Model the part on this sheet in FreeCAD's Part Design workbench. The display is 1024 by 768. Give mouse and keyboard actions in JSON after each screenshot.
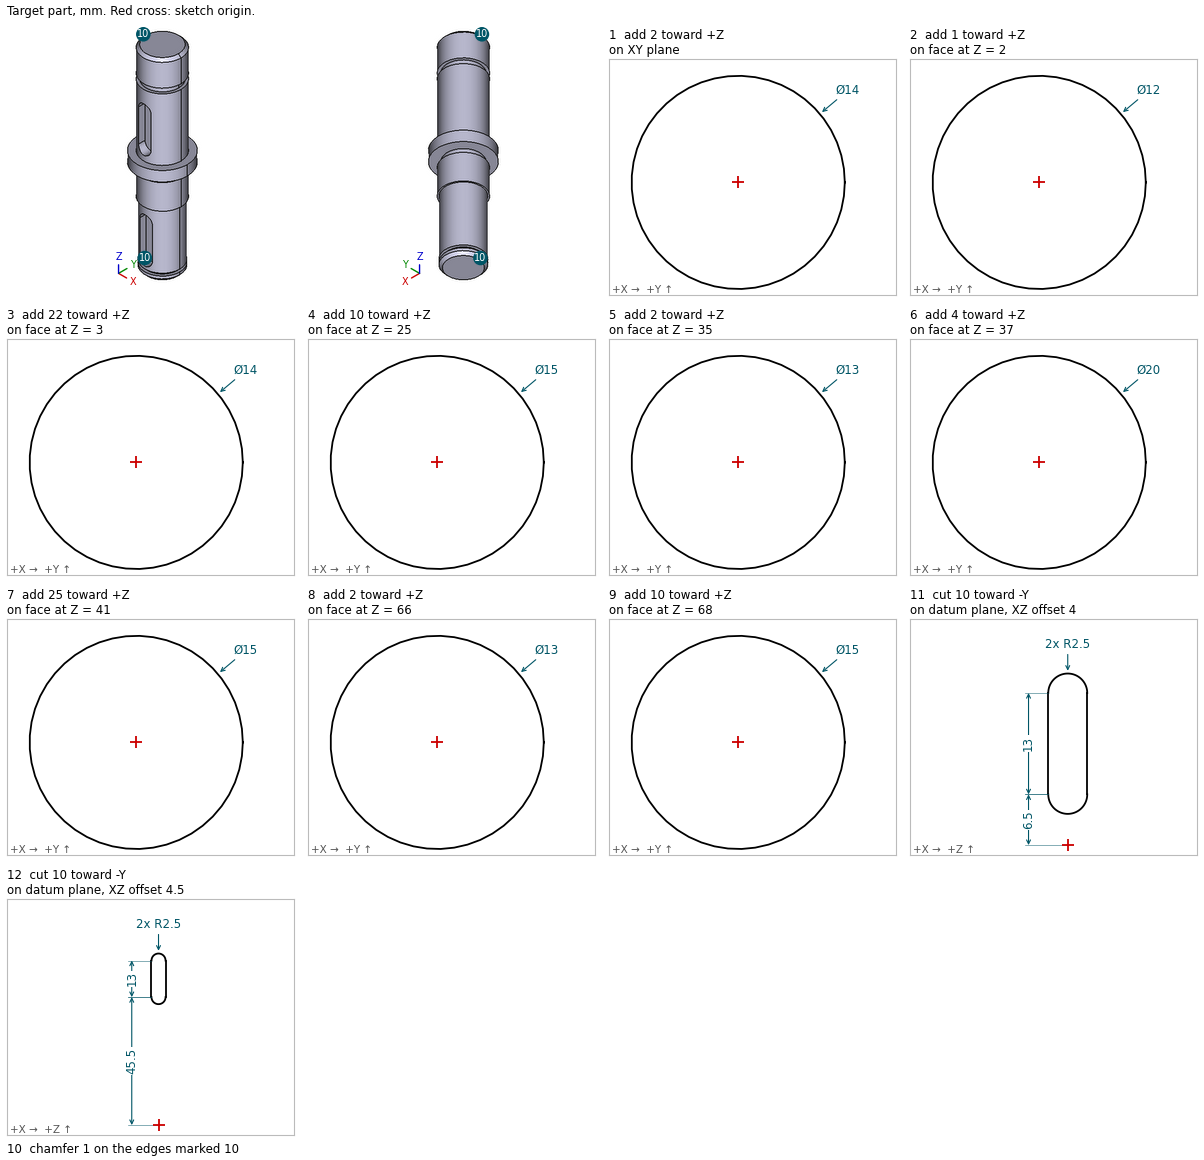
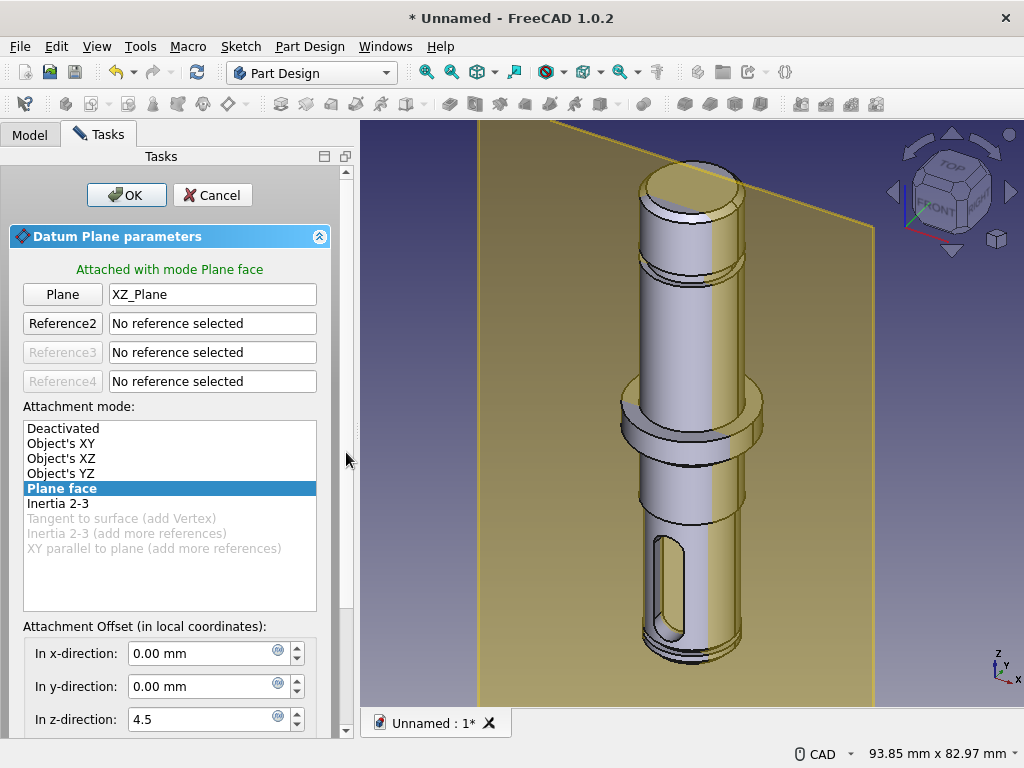
{"action": "left_click", "coordinate": [127, 195]}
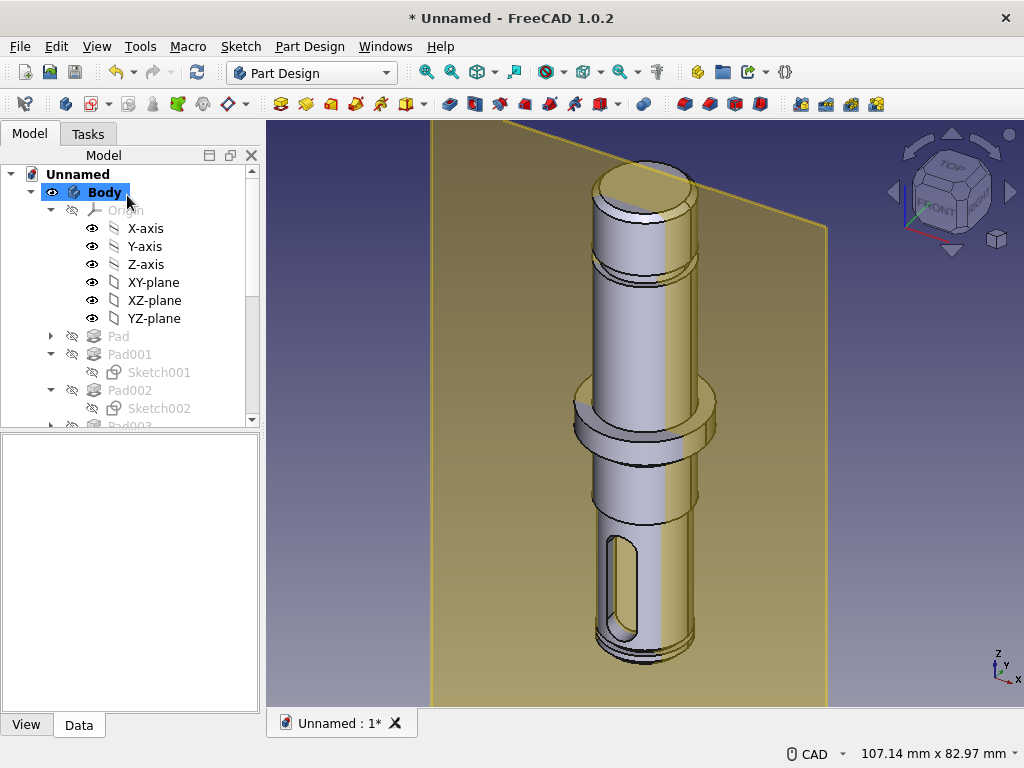
{"action": "scroll", "coordinate": [101, 296], "scroll_direction": "down", "scroll_amount": 3}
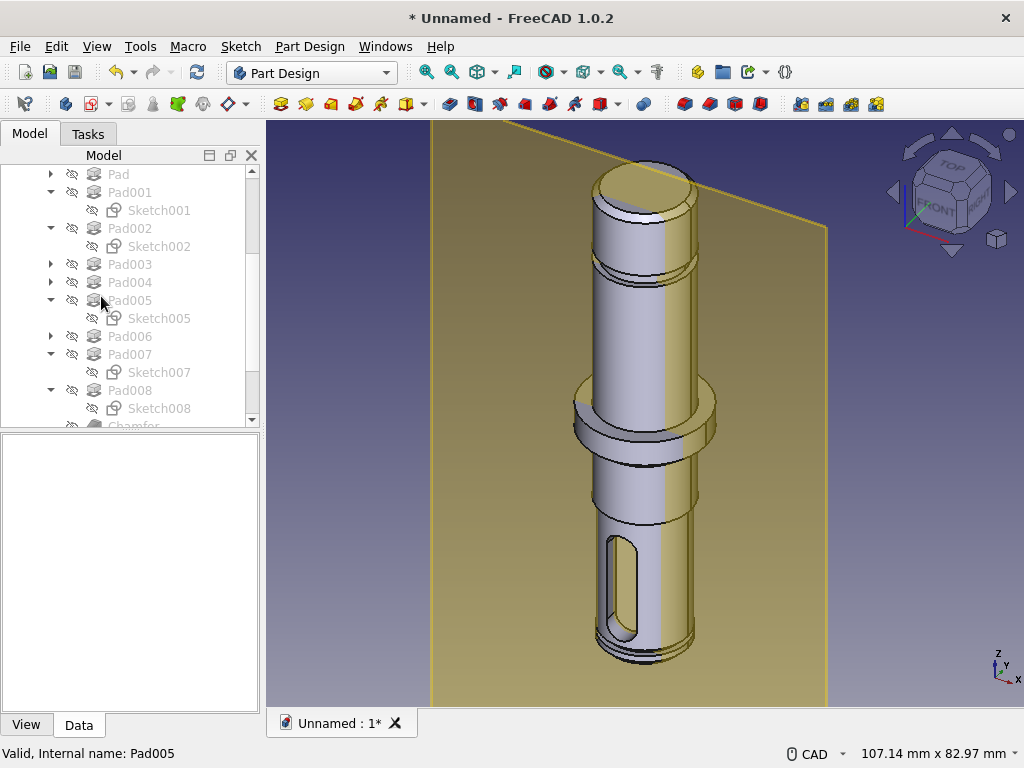
{"action": "scroll", "coordinate": [141, 296], "scroll_direction": "up", "scroll_amount": 15}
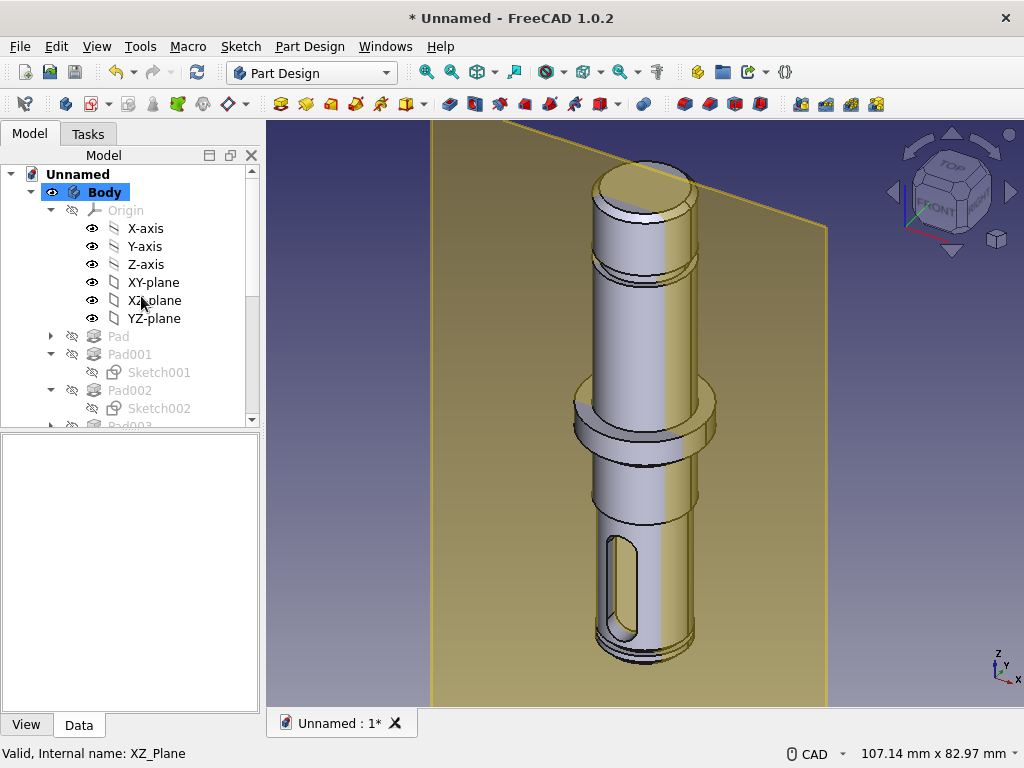
{"action": "scroll", "coordinate": [101, 296], "scroll_direction": "down", "scroll_amount": 6}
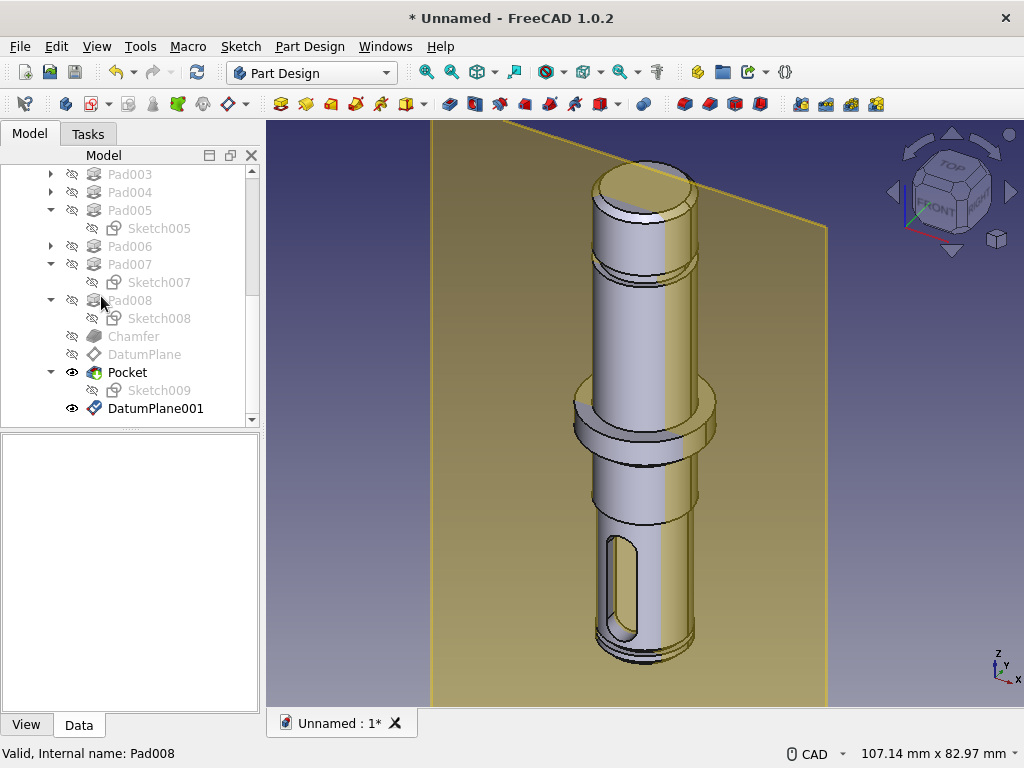
{"action": "left_click", "coordinate": [117, 408]}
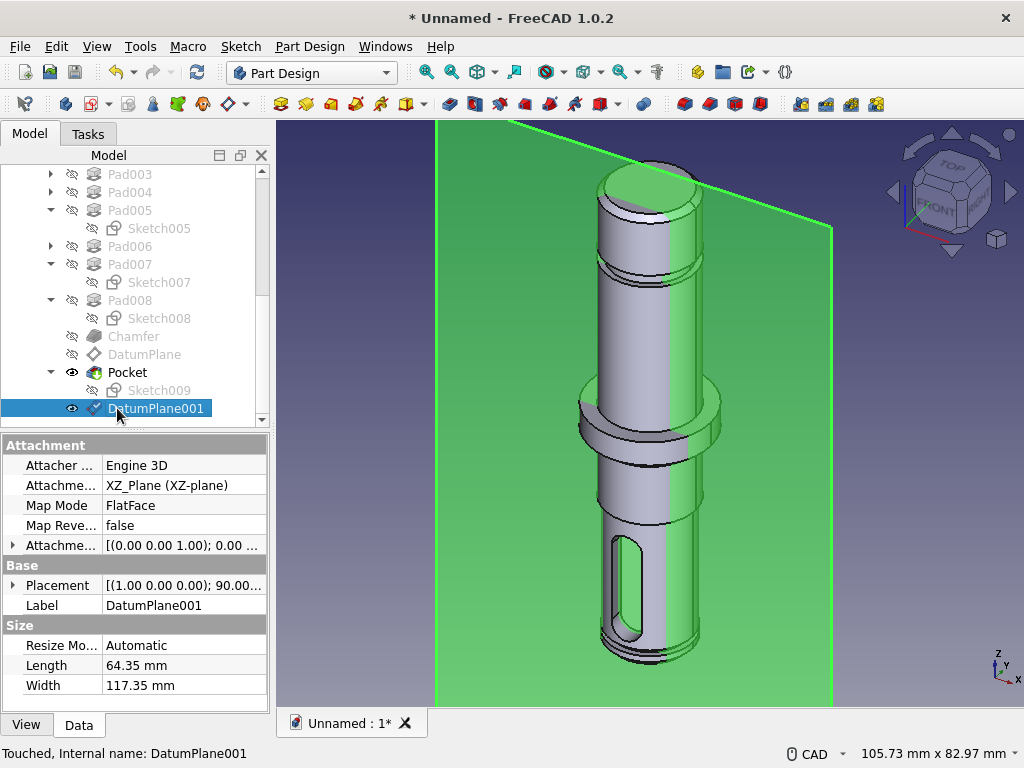
{"action": "left_click", "coordinate": [90, 104]}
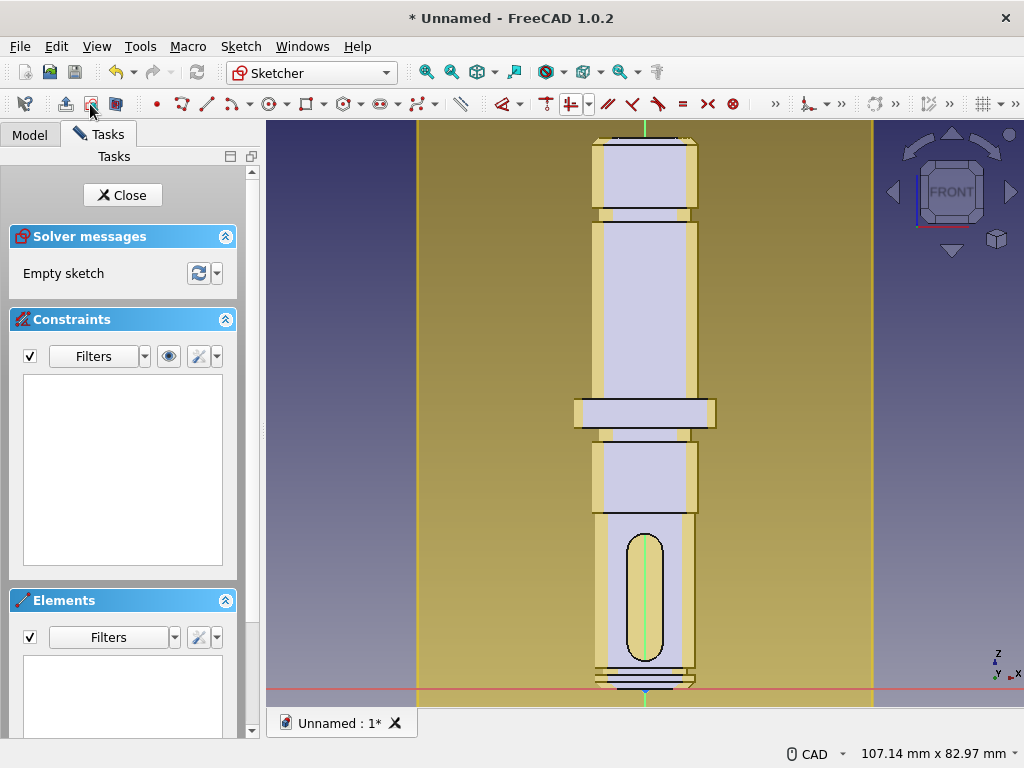
{"action": "left_click", "coordinate": [116, 104]}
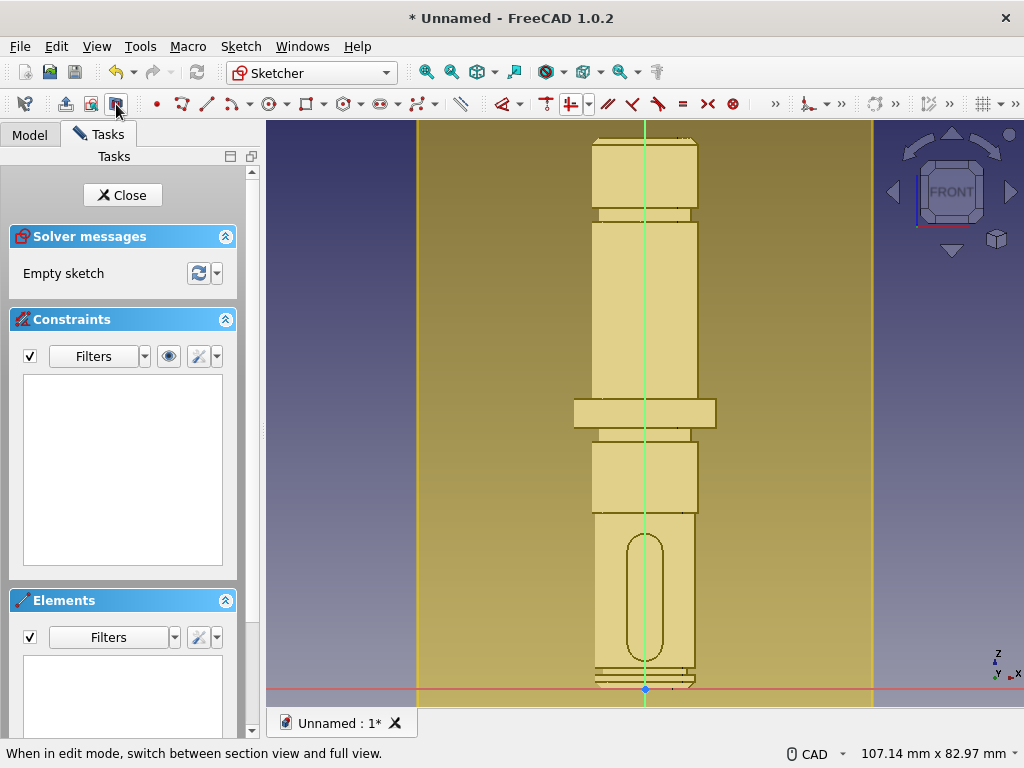
{"action": "scroll", "coordinate": [685, 268], "scroll_direction": "up", "scroll_amount": 5}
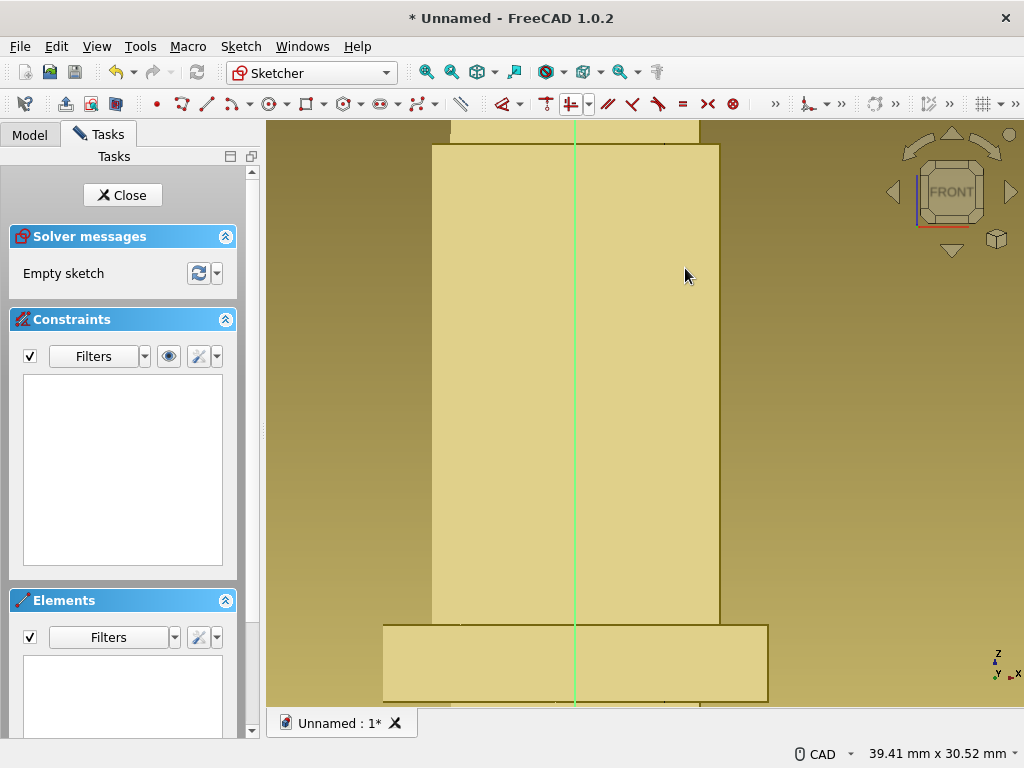
{"action": "left_click", "coordinate": [380, 104]}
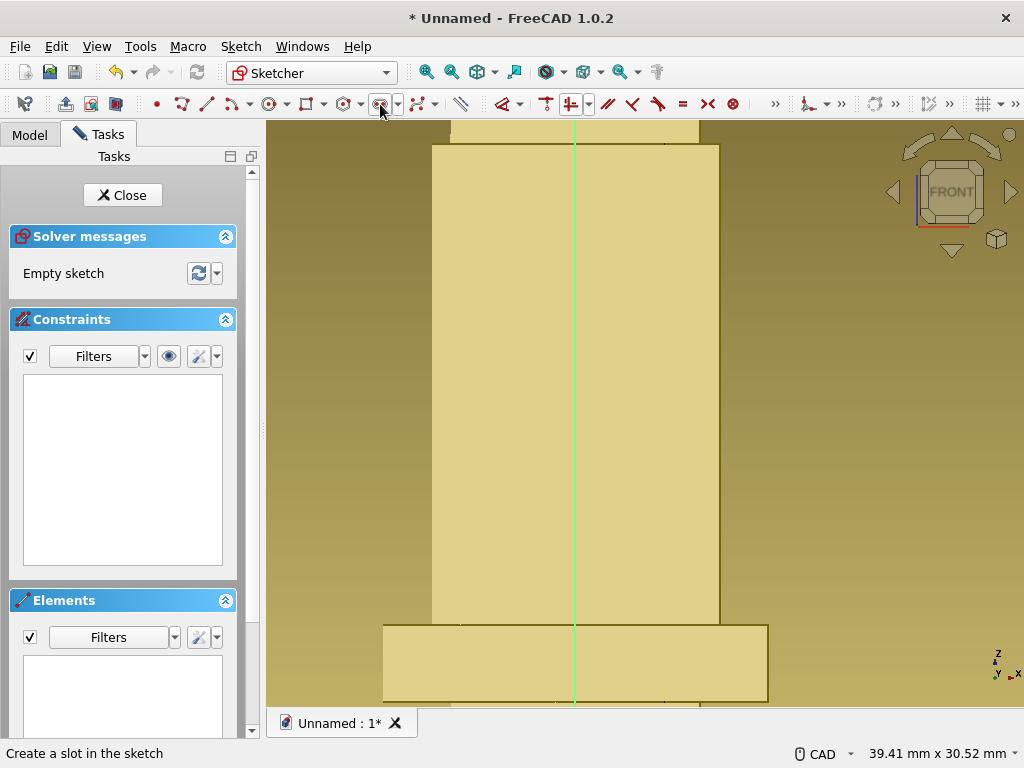
{"action": "left_click", "coordinate": [575, 538]}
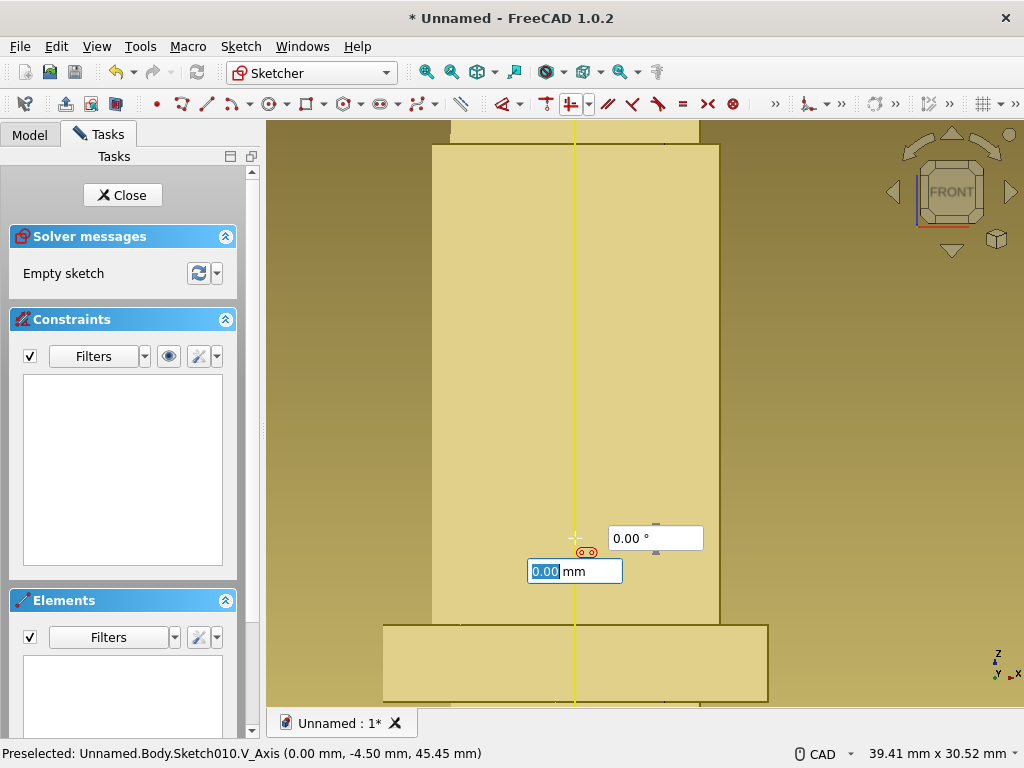
{"action": "left_click", "coordinate": [584, 288]}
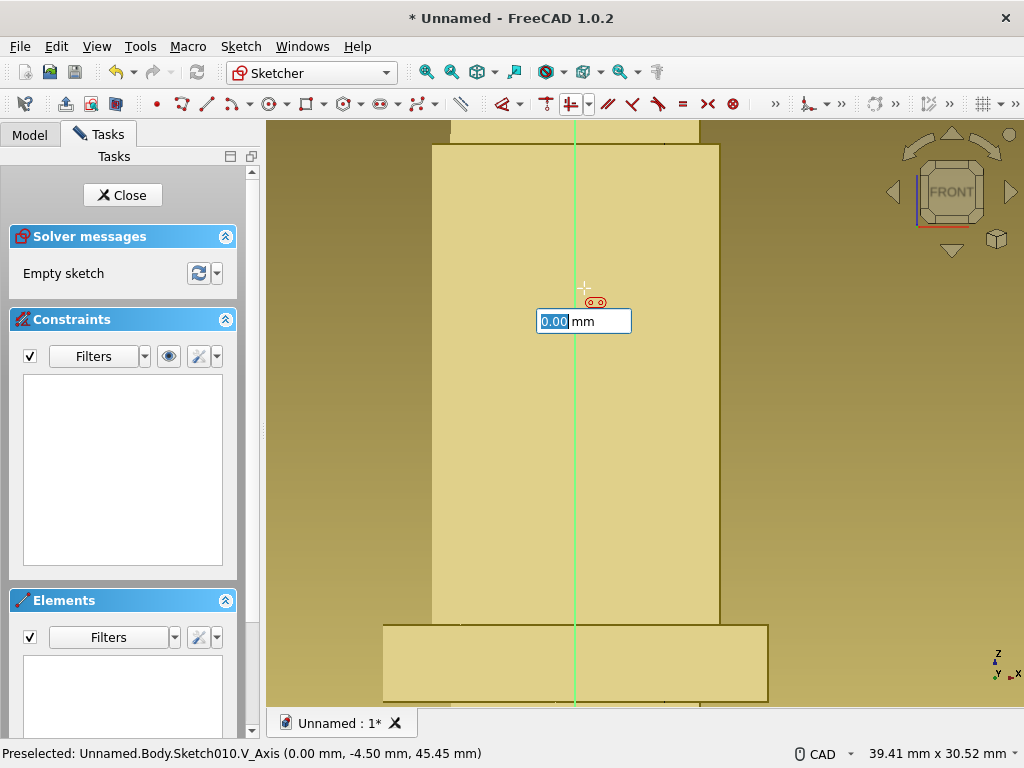
{"action": "left_click", "coordinate": [623, 413]}
{"action": "key", "text": "Escape"}